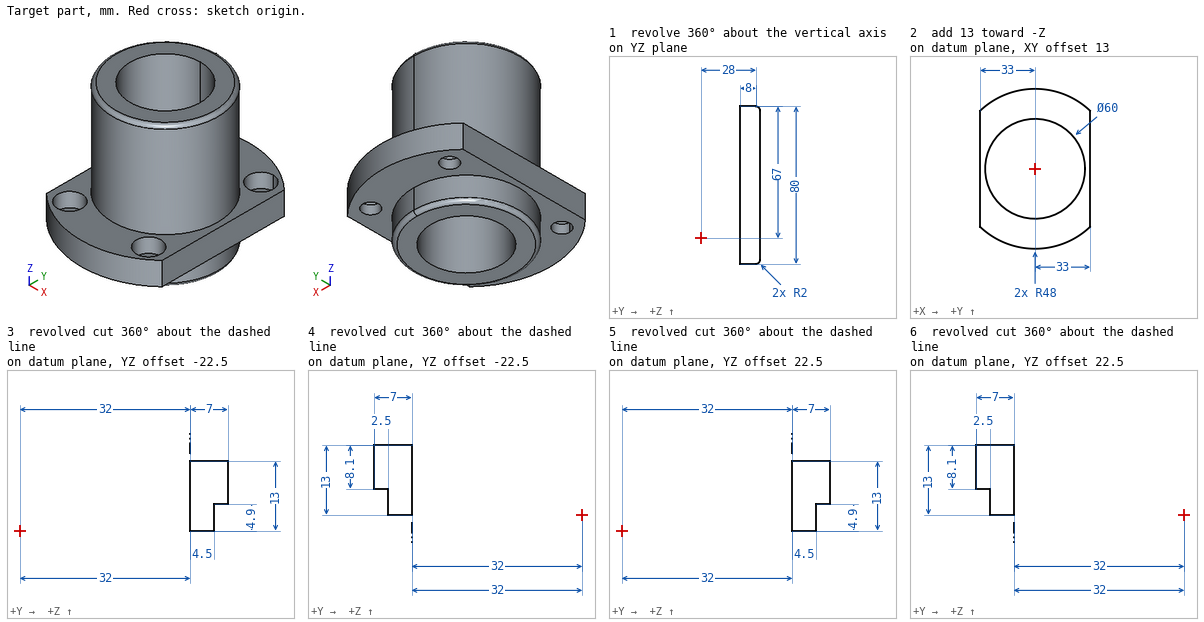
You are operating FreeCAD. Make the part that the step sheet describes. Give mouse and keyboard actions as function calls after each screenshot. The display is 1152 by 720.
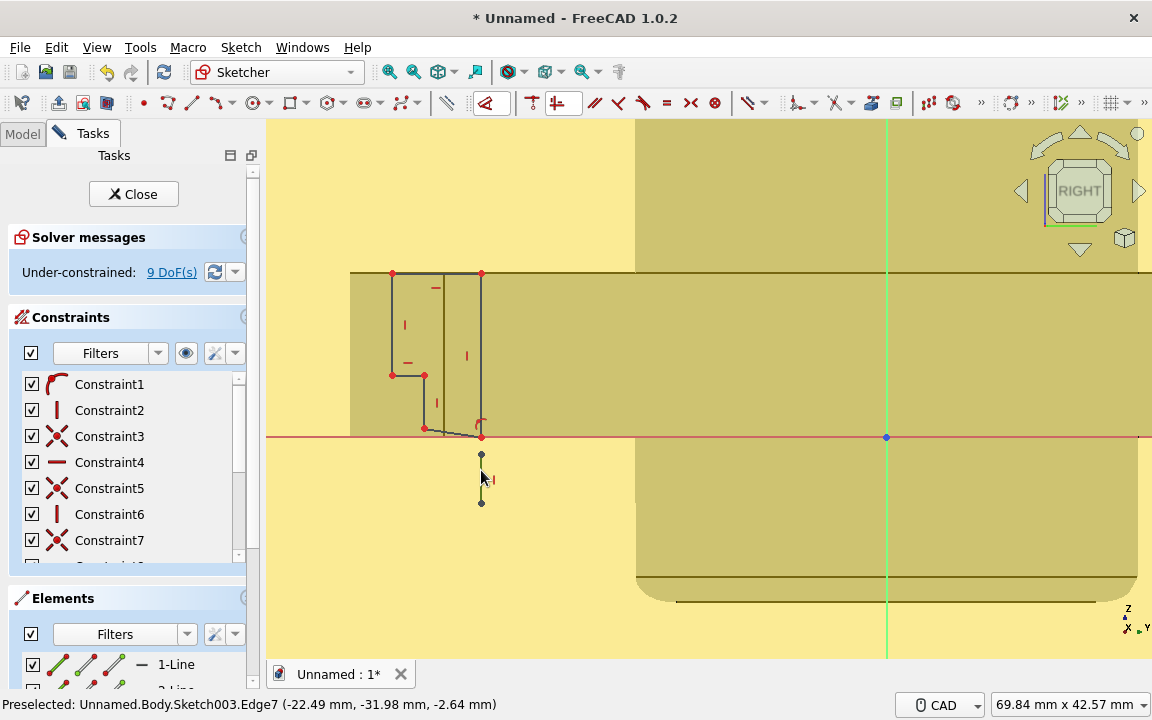
click(448, 104)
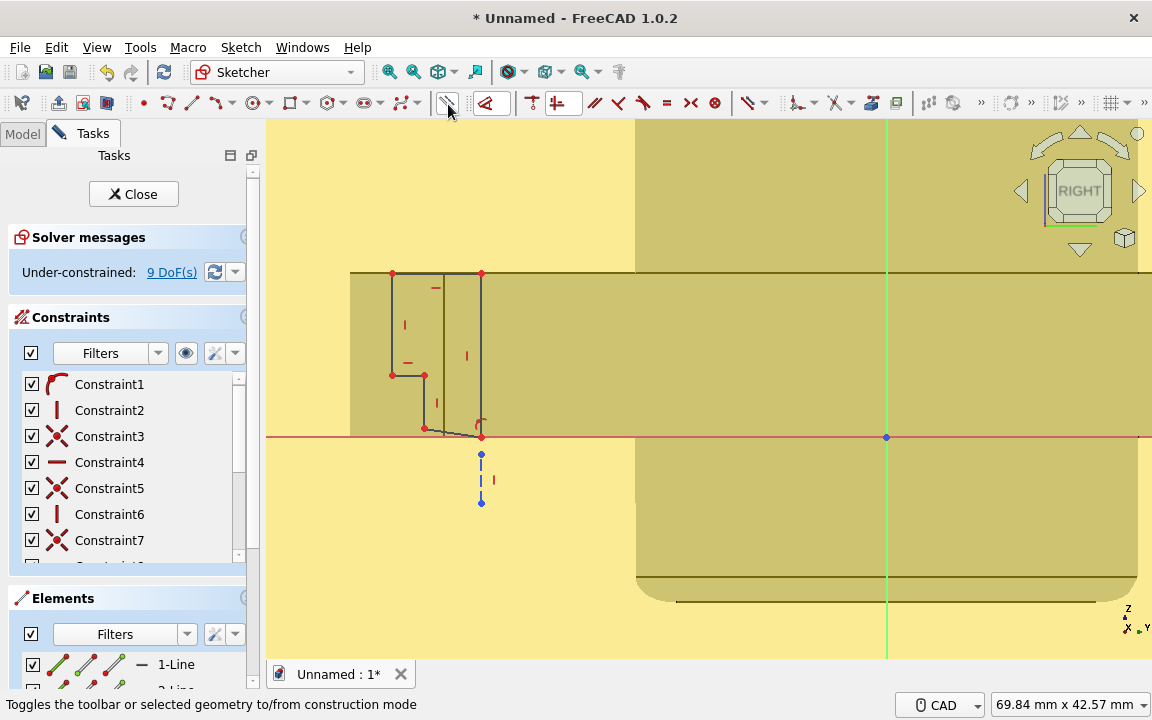
click(464, 435)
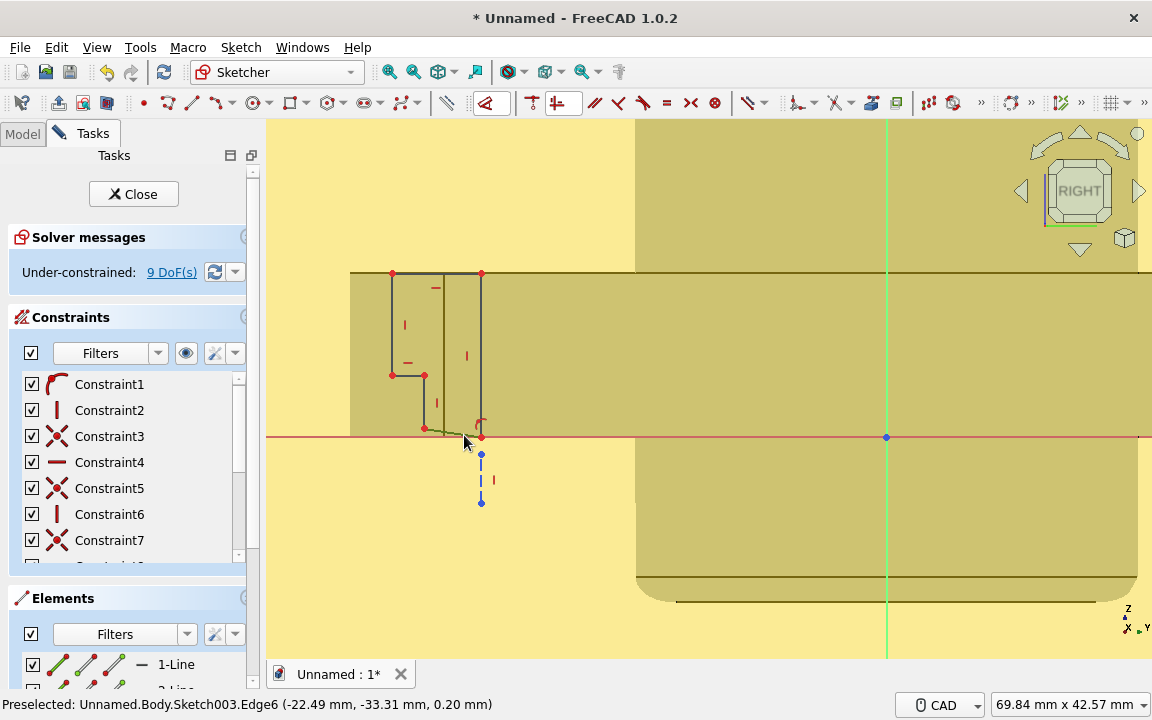
key(h)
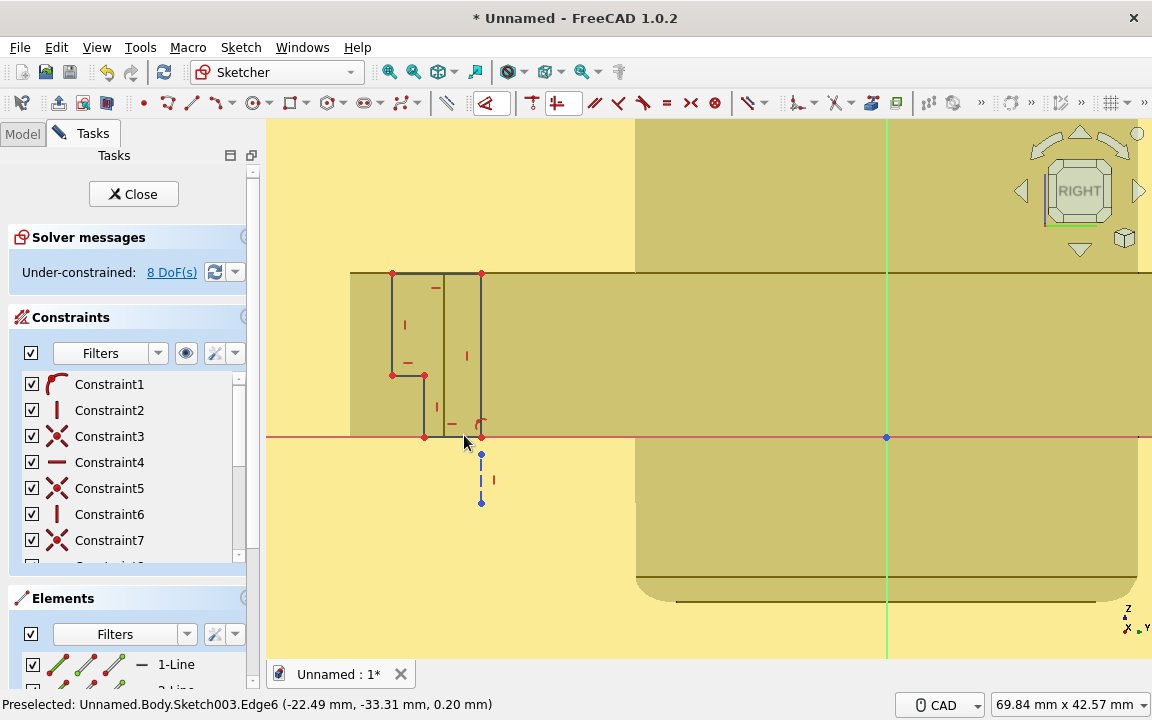
click(454, 274)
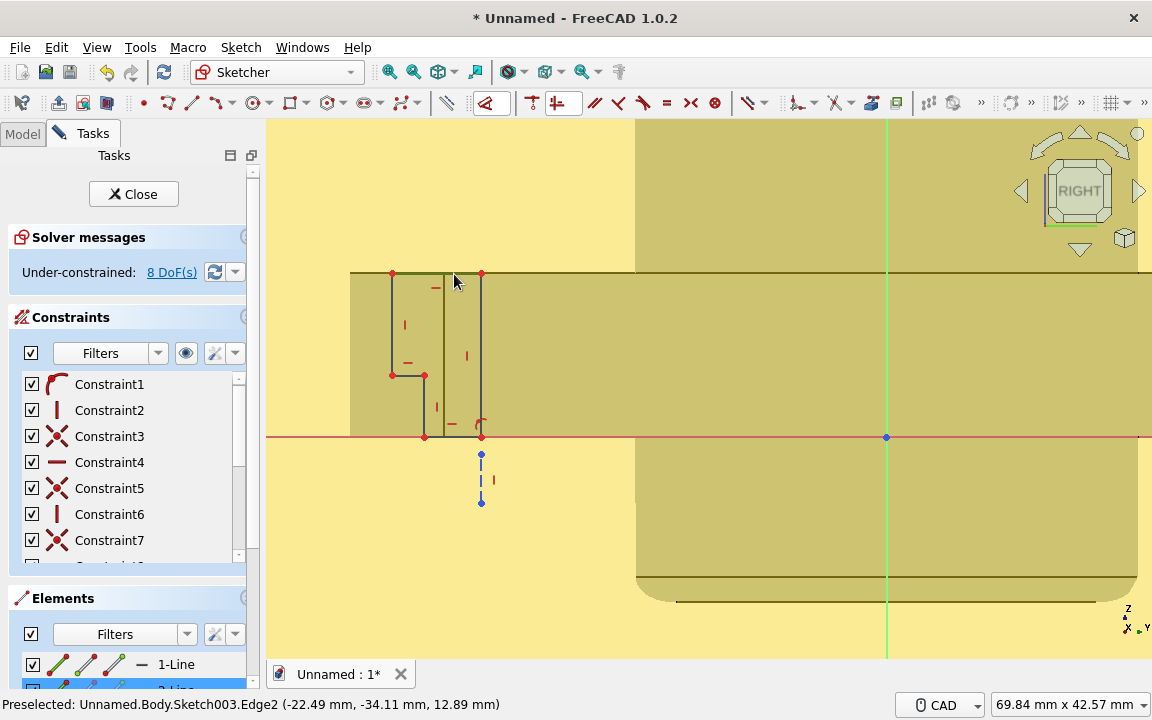
key(l)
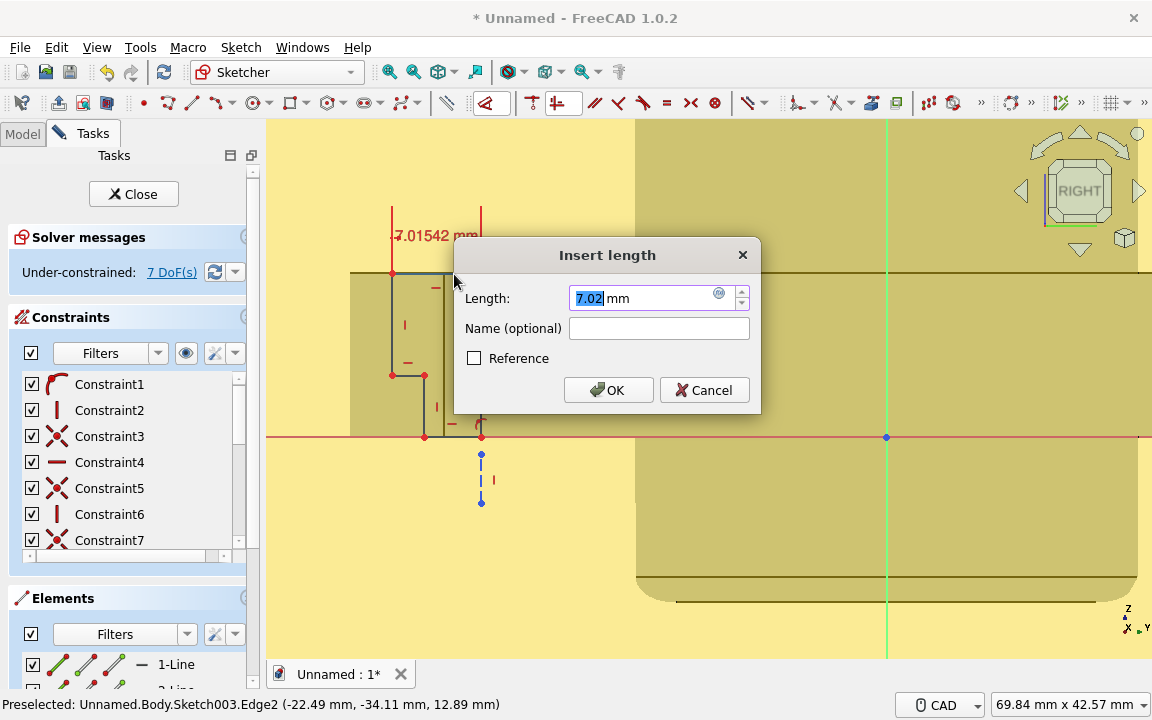
text(7)
key(Return)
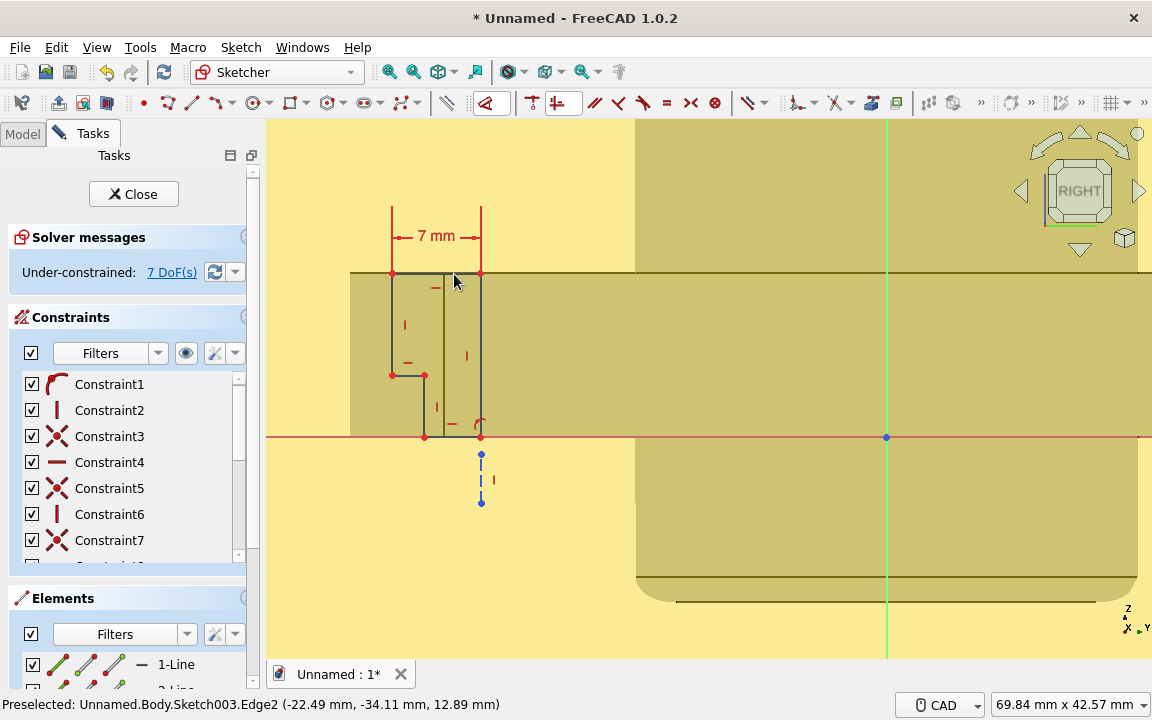
click(481, 388)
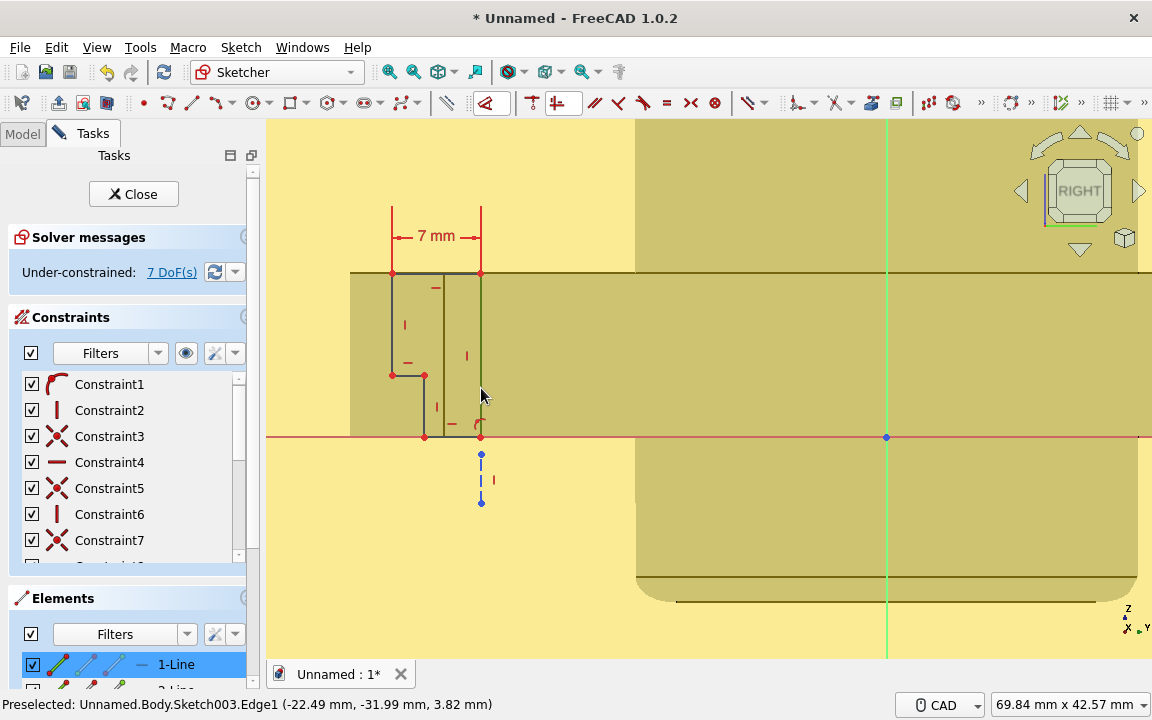
key(i)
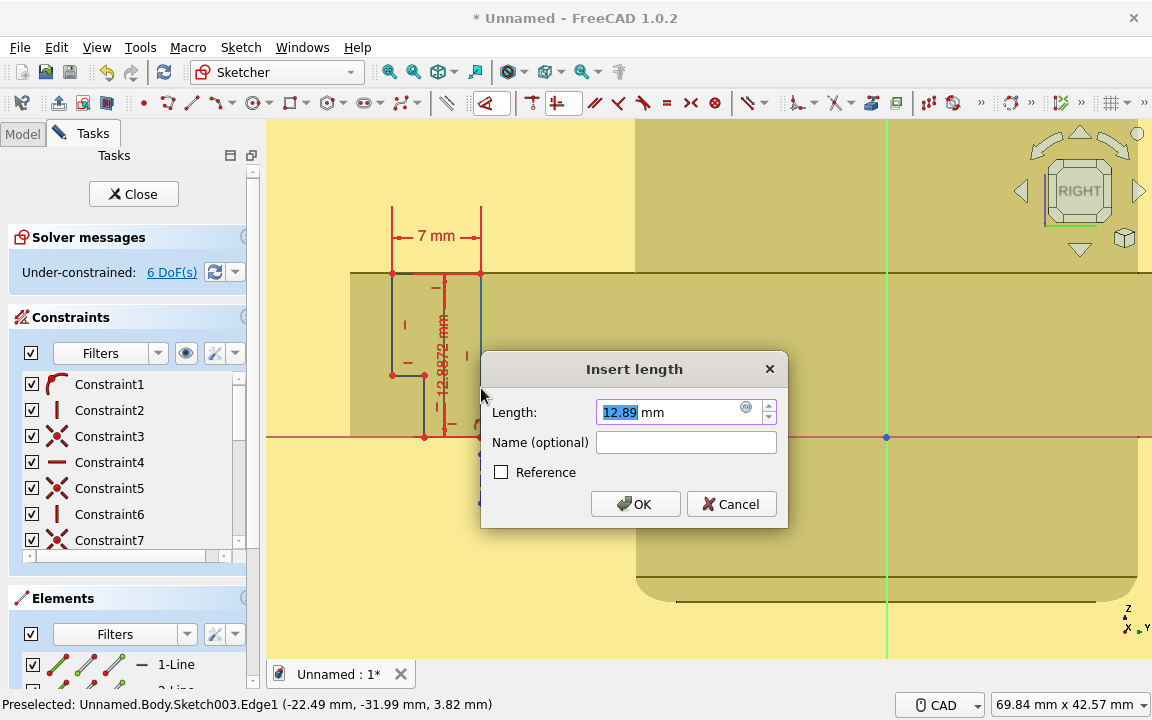
text(13)
key(Return)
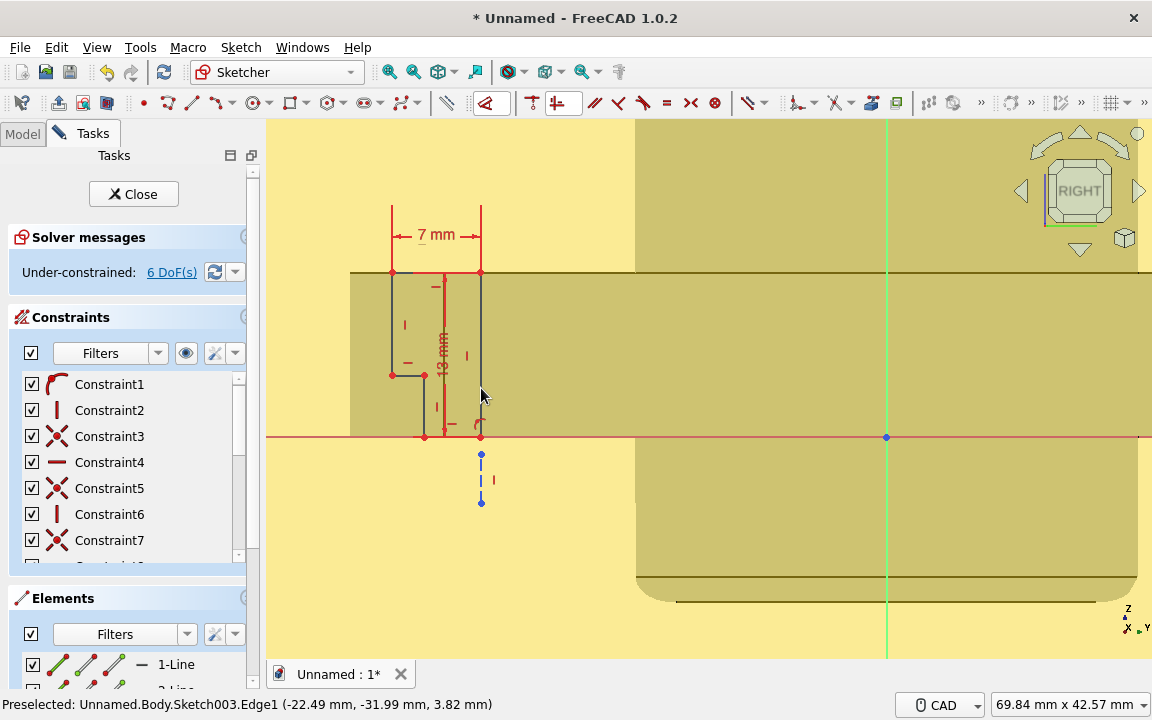
click(392, 304)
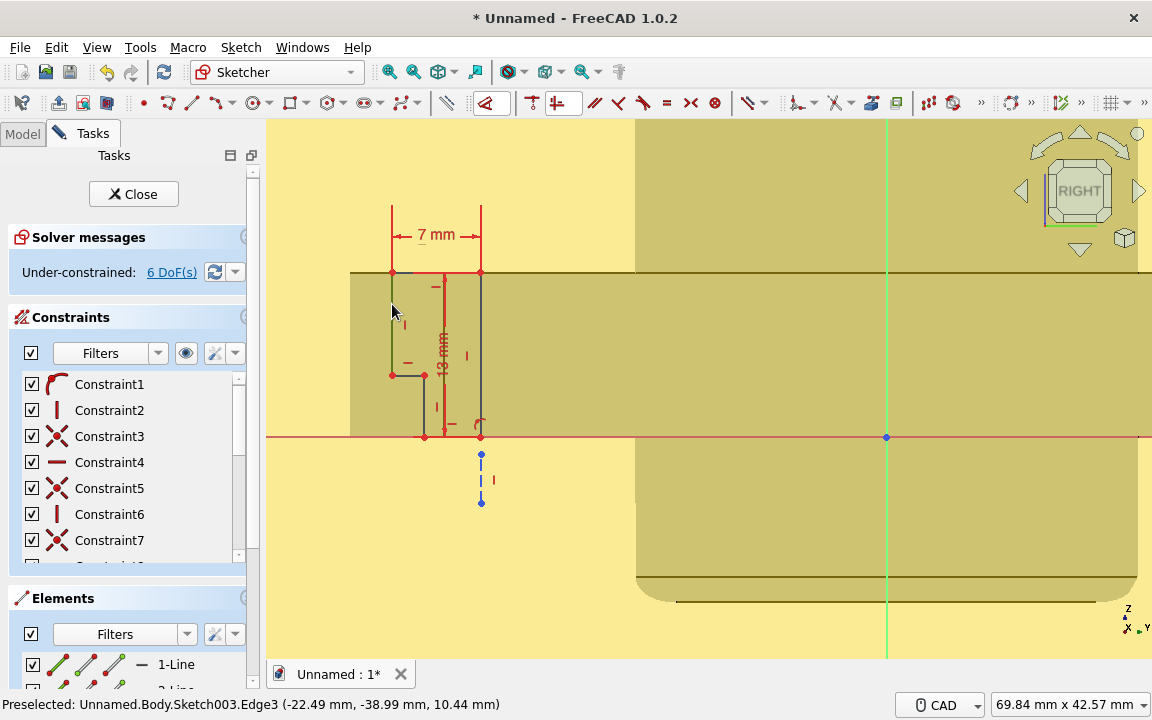
key(i)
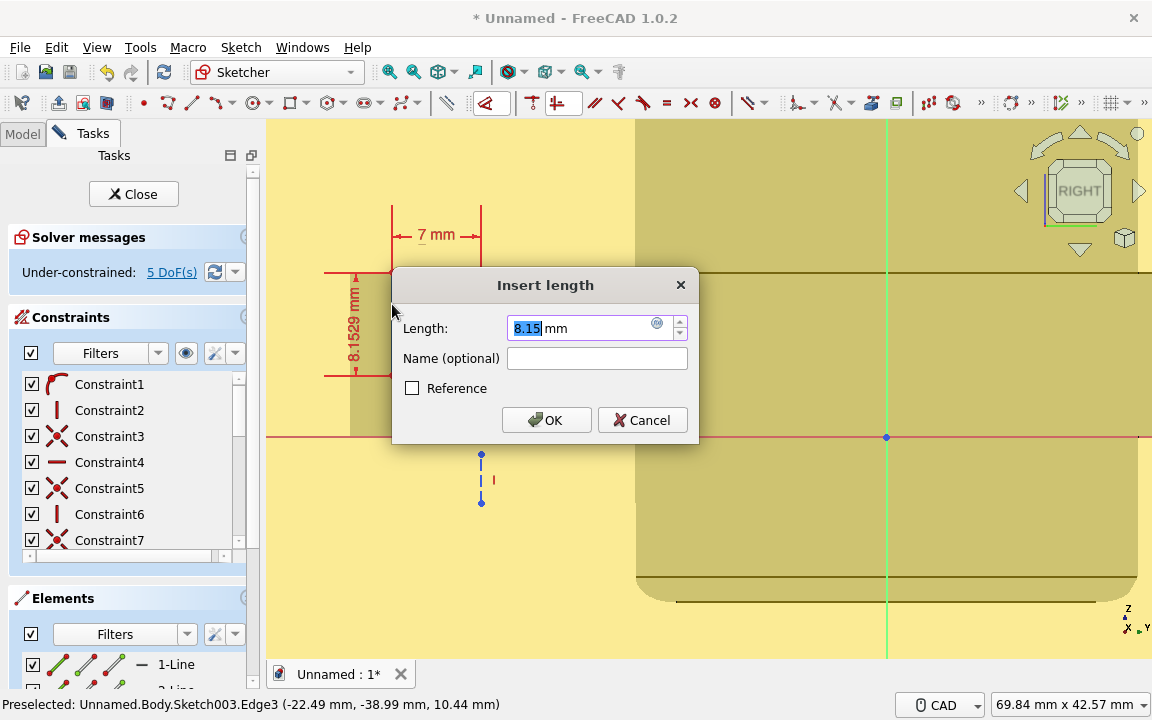
text(8.1)
key(Return)